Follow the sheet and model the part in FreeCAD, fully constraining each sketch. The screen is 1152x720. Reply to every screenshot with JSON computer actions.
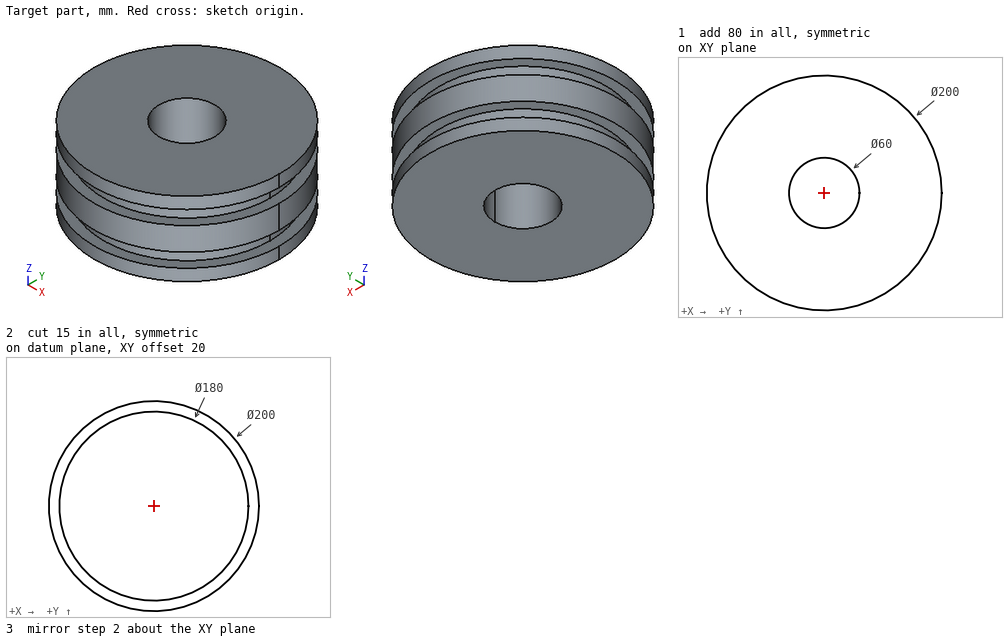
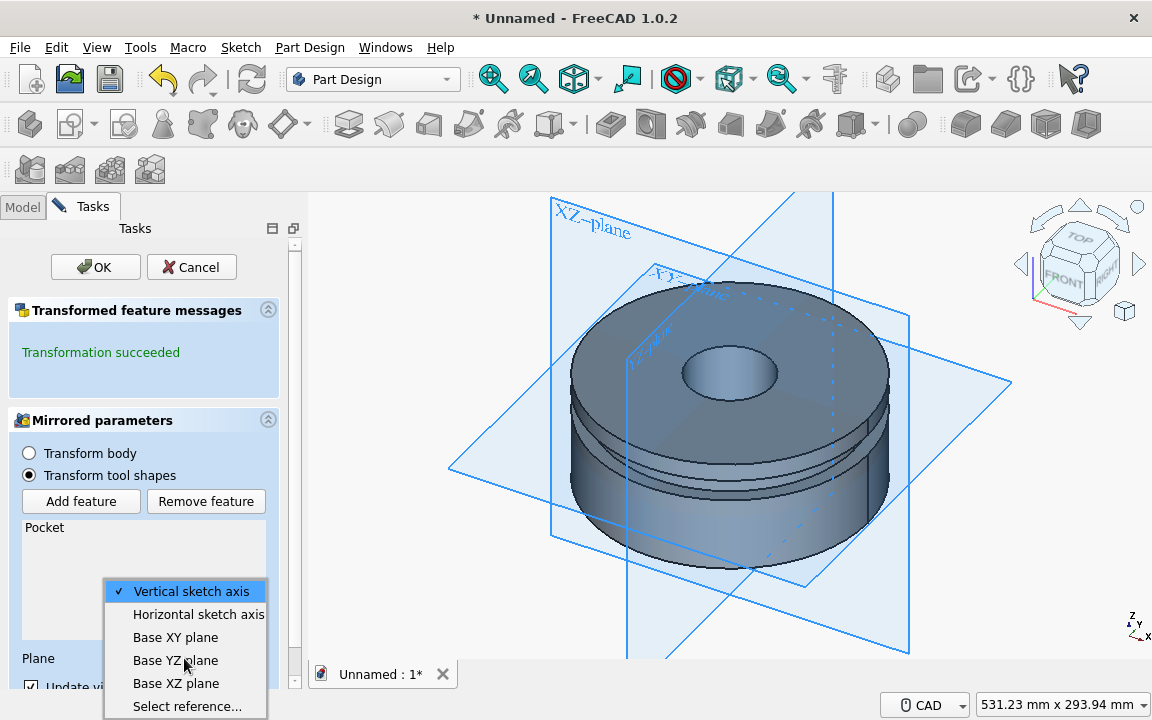
{"action": "left_click", "coordinate": [184, 638]}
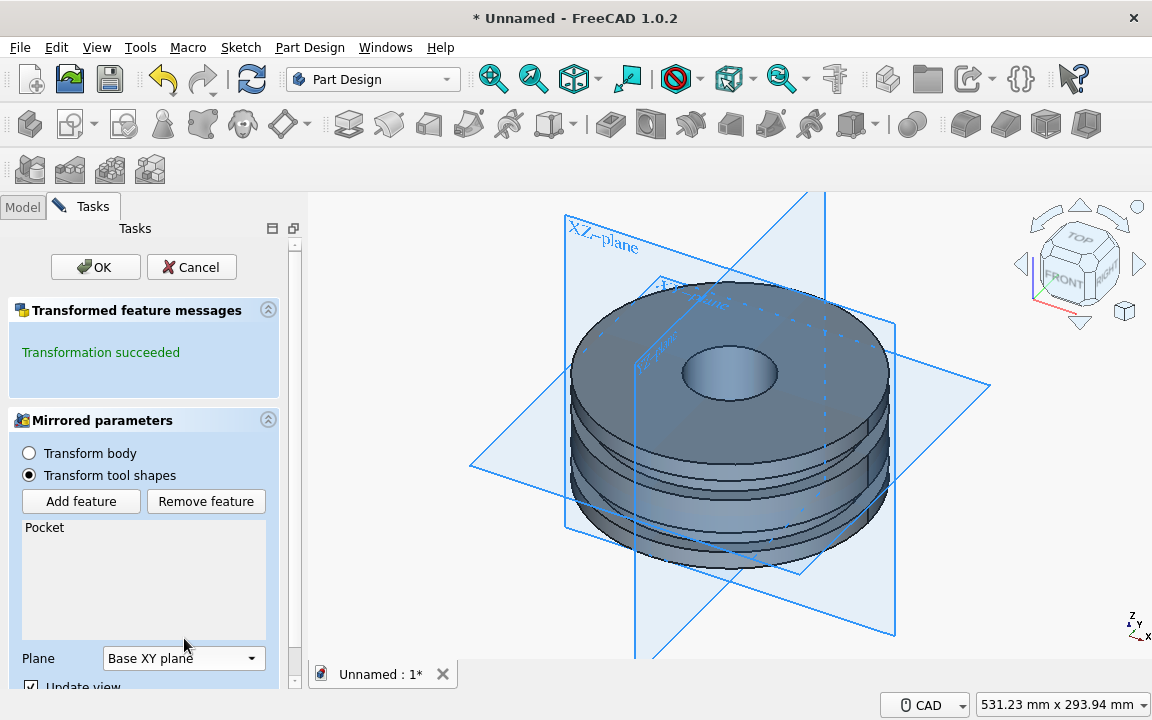
{"action": "left_click", "coordinate": [96, 267]}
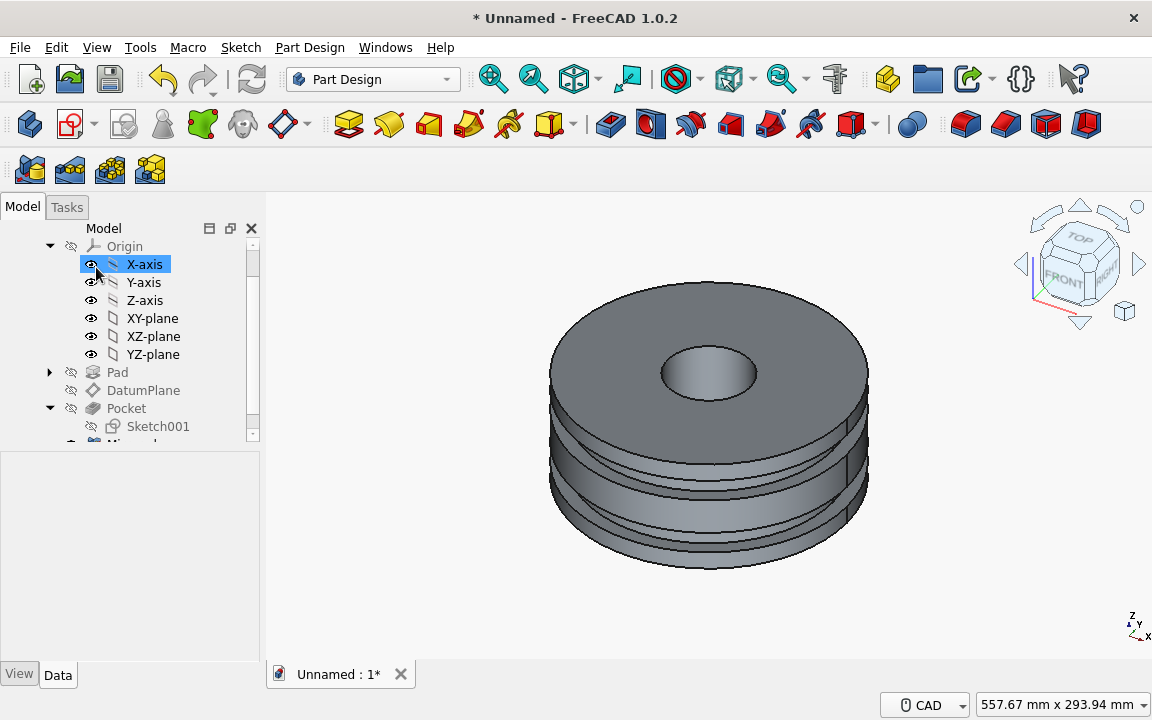
{"action": "key", "text": "0"}